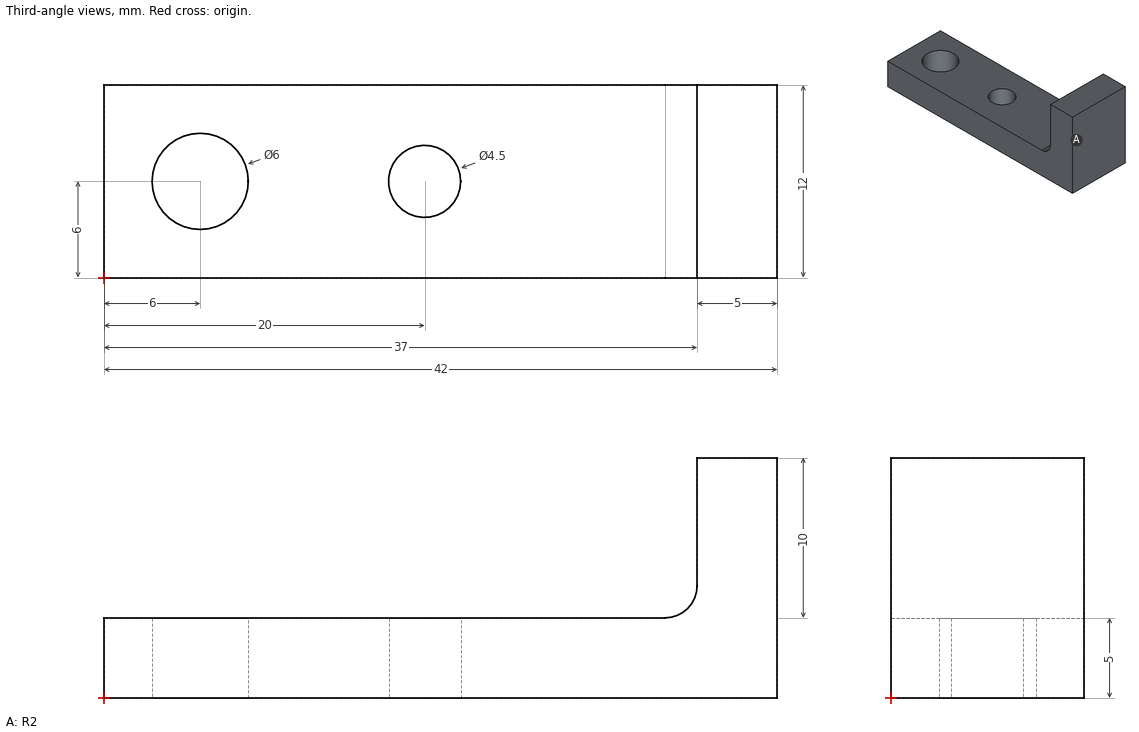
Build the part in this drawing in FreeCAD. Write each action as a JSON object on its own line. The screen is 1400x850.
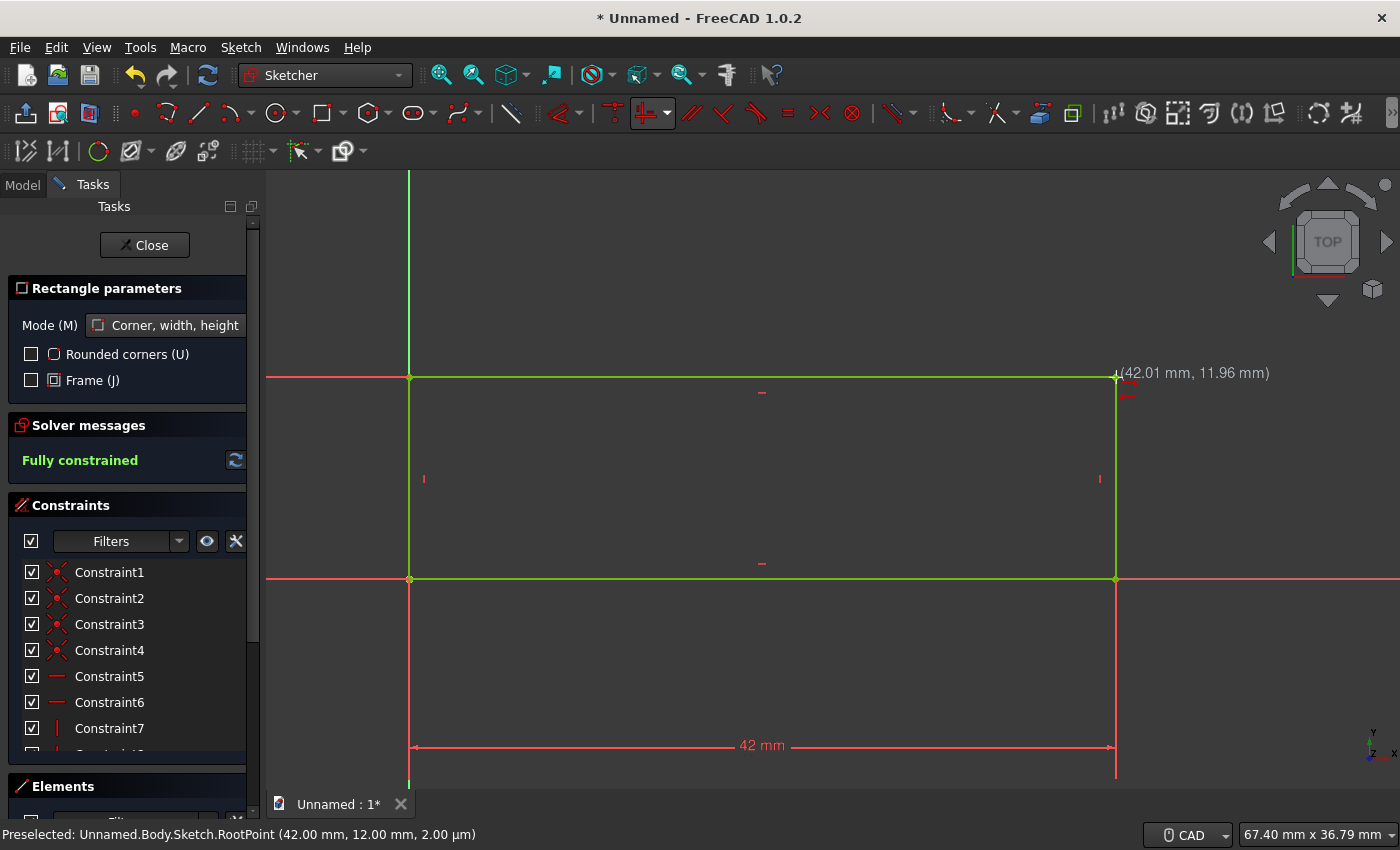
{"action": "left_click", "coordinate": [276, 114]}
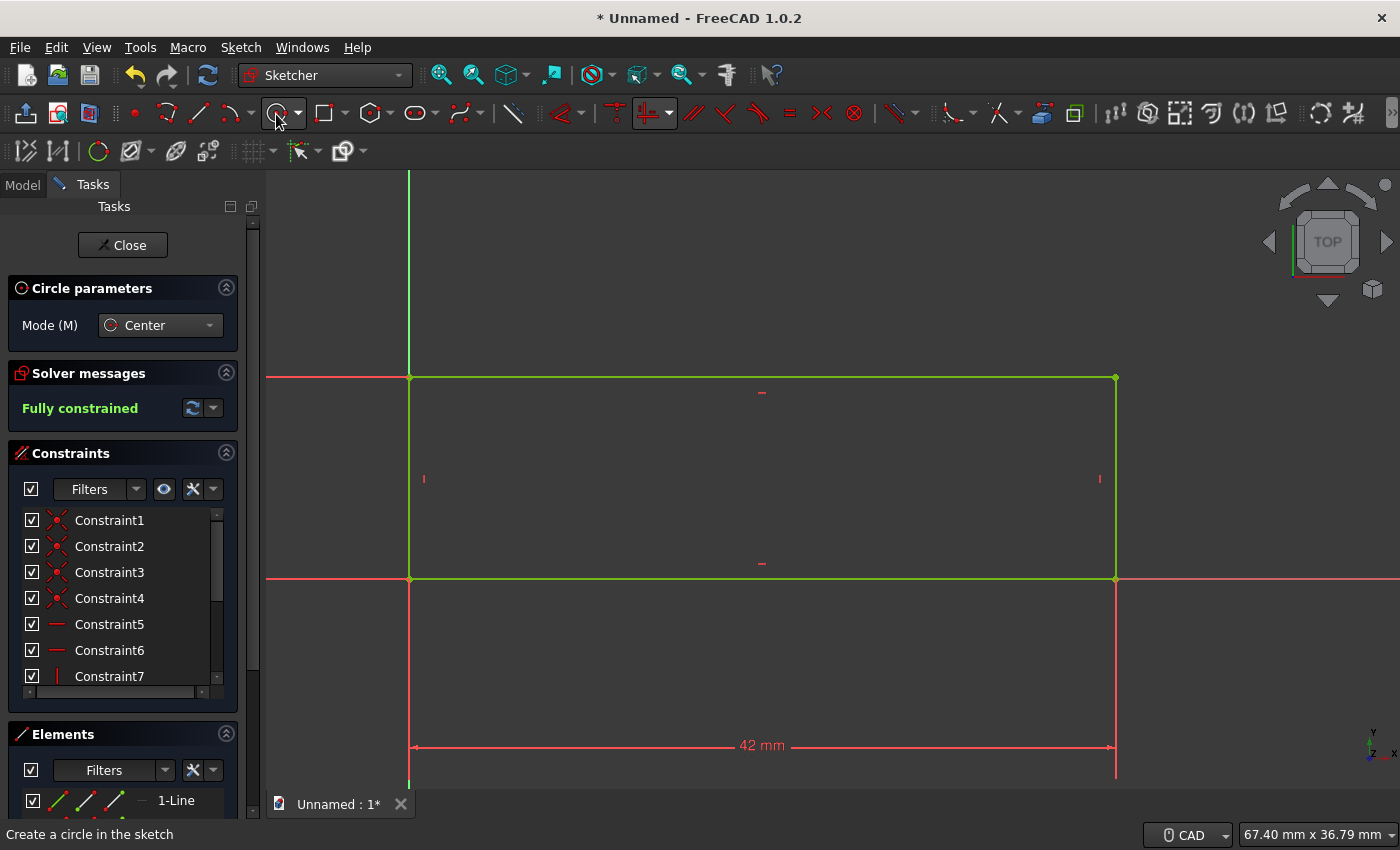
{"action": "left_click", "coordinate": [510, 478]}
{"action": "mouse_move", "coordinate": [546, 443]}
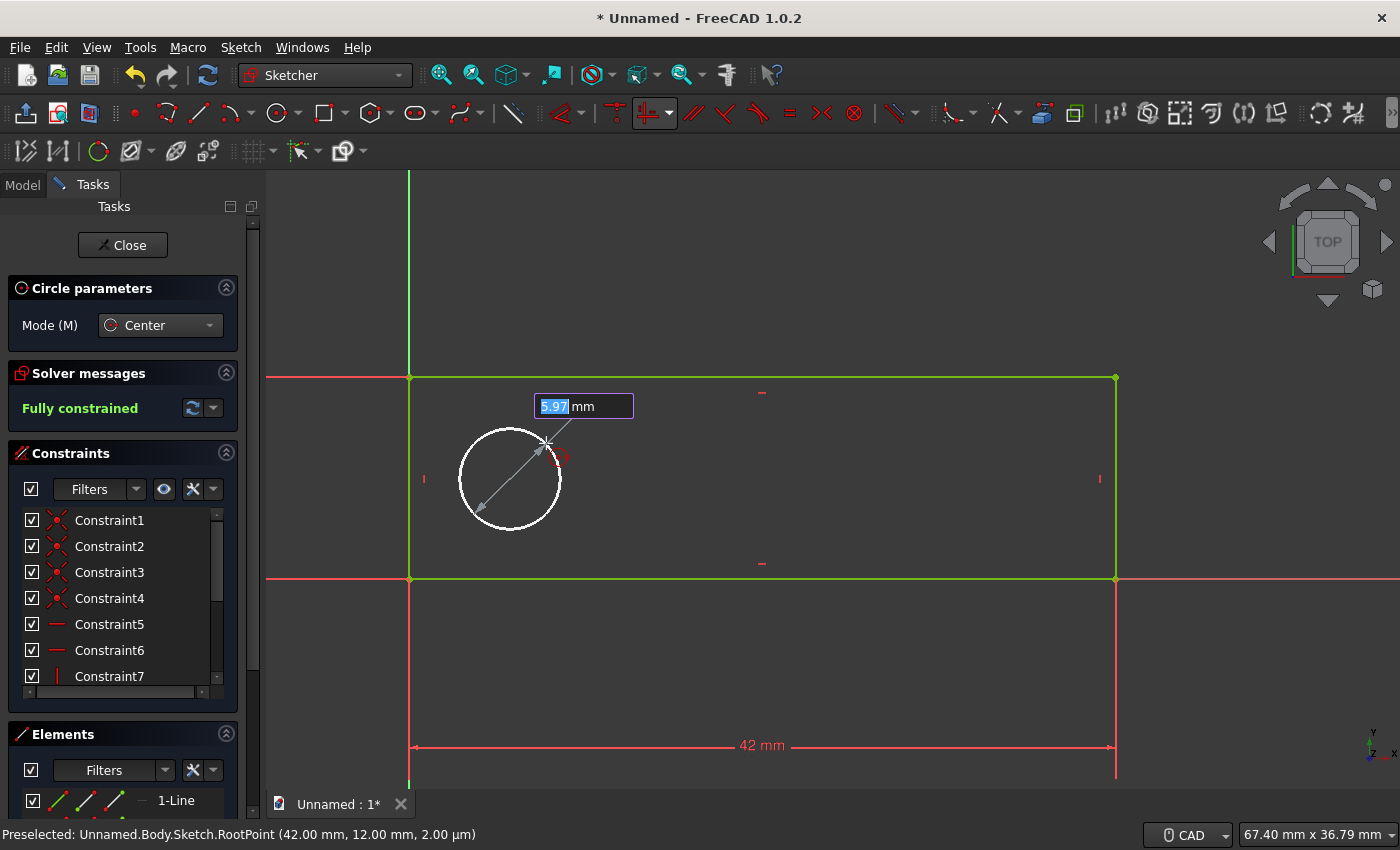
{"action": "type", "text": "6"}
{"action": "key", "text": "Return"}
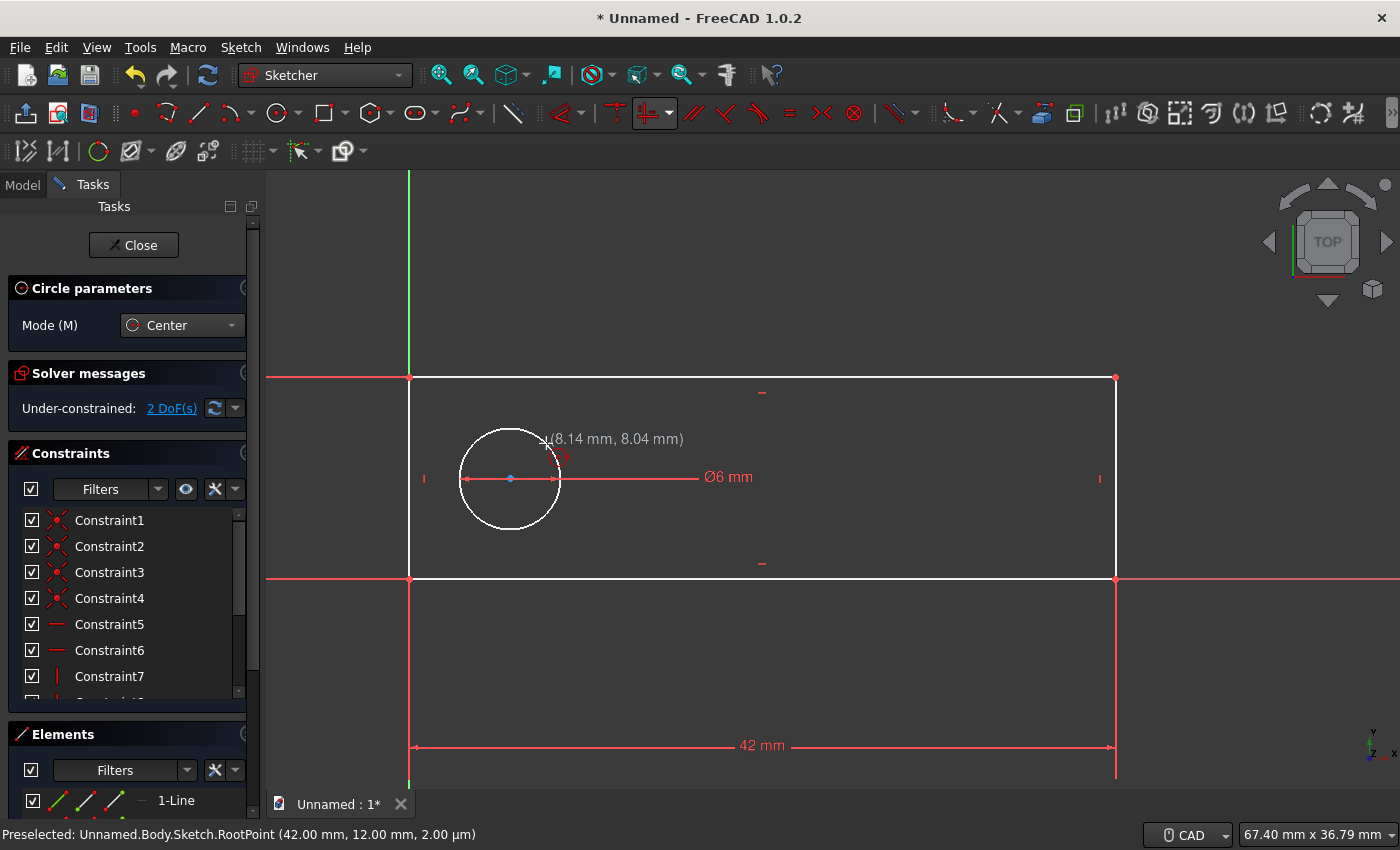
{"action": "left_click", "coordinate": [746, 478]}
{"action": "mouse_move", "coordinate": [772, 452]}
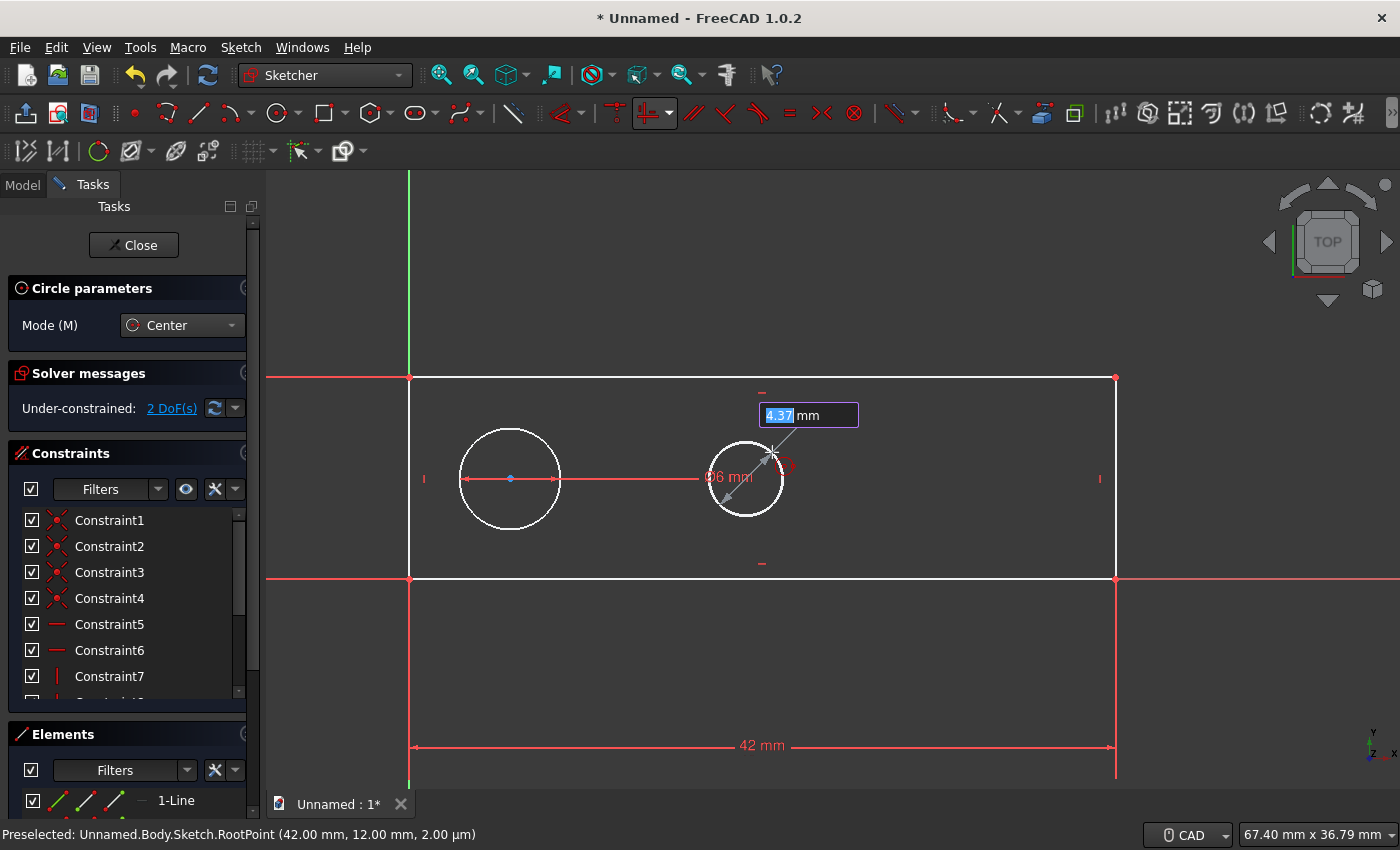
{"action": "type", "text": "4.5"}
{"action": "key", "text": "Return"}
{"action": "key", "text": "Escape"}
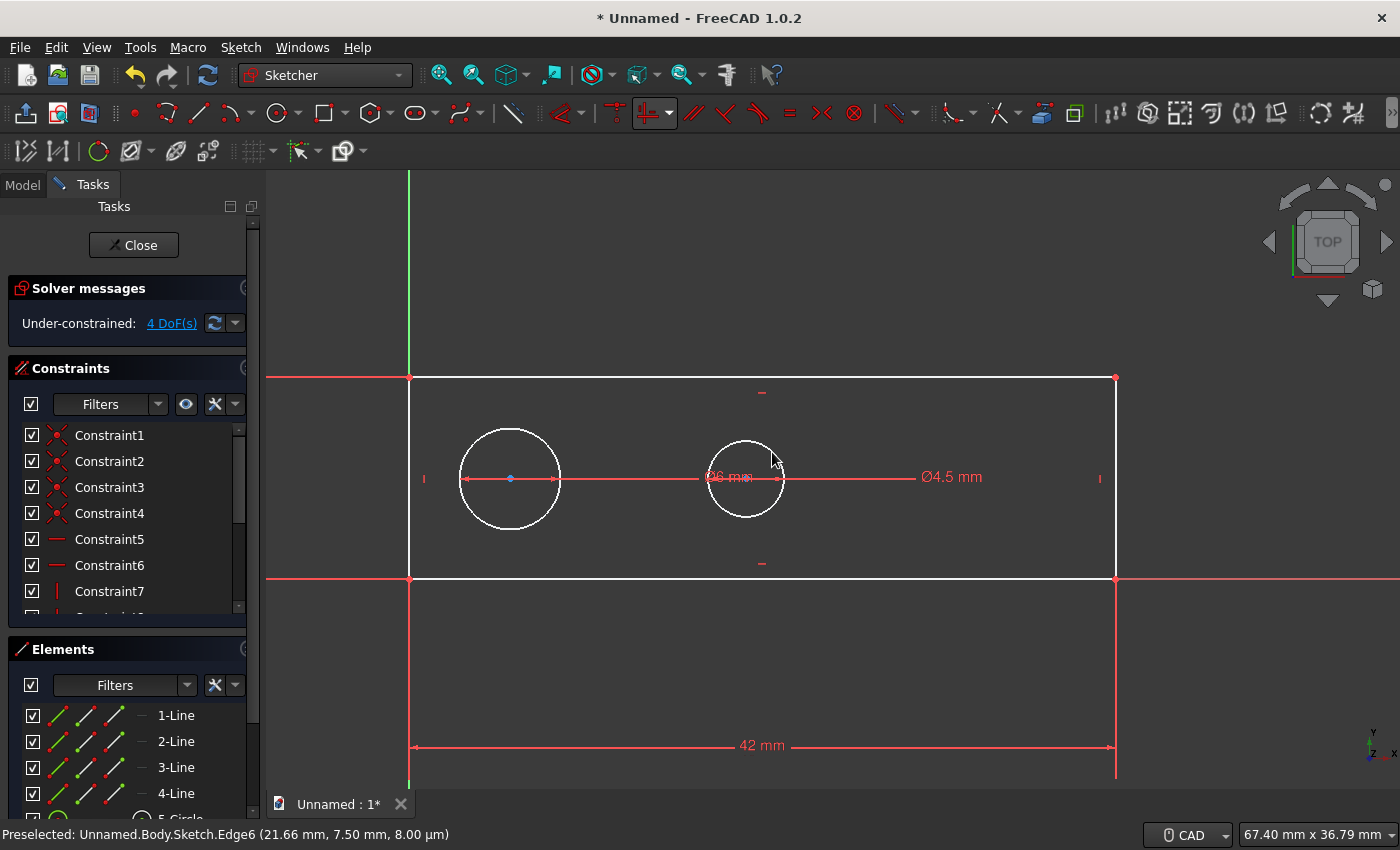
{"action": "left_click", "coordinate": [510, 479]}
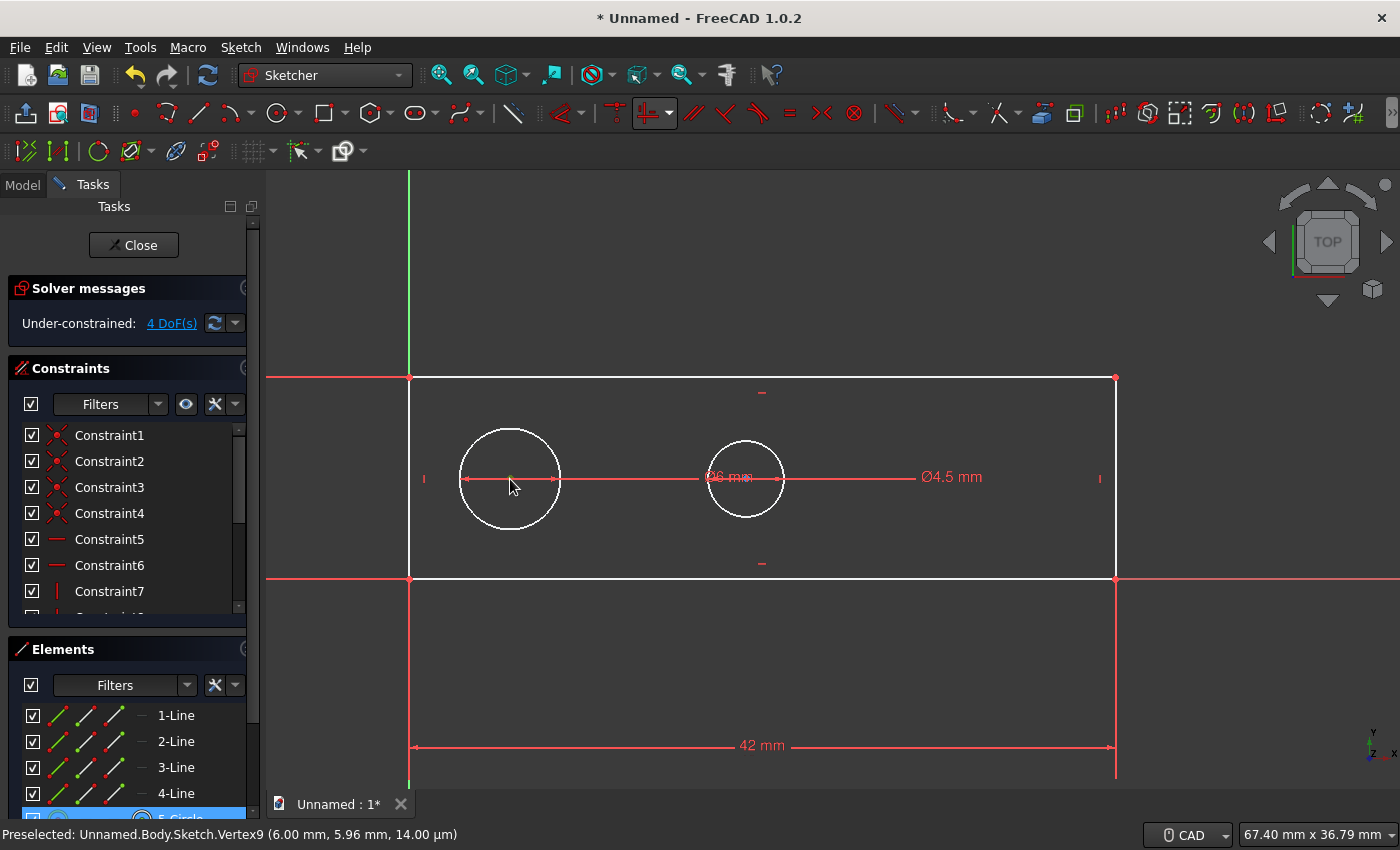
{"action": "left_click", "coordinate": [746, 479]}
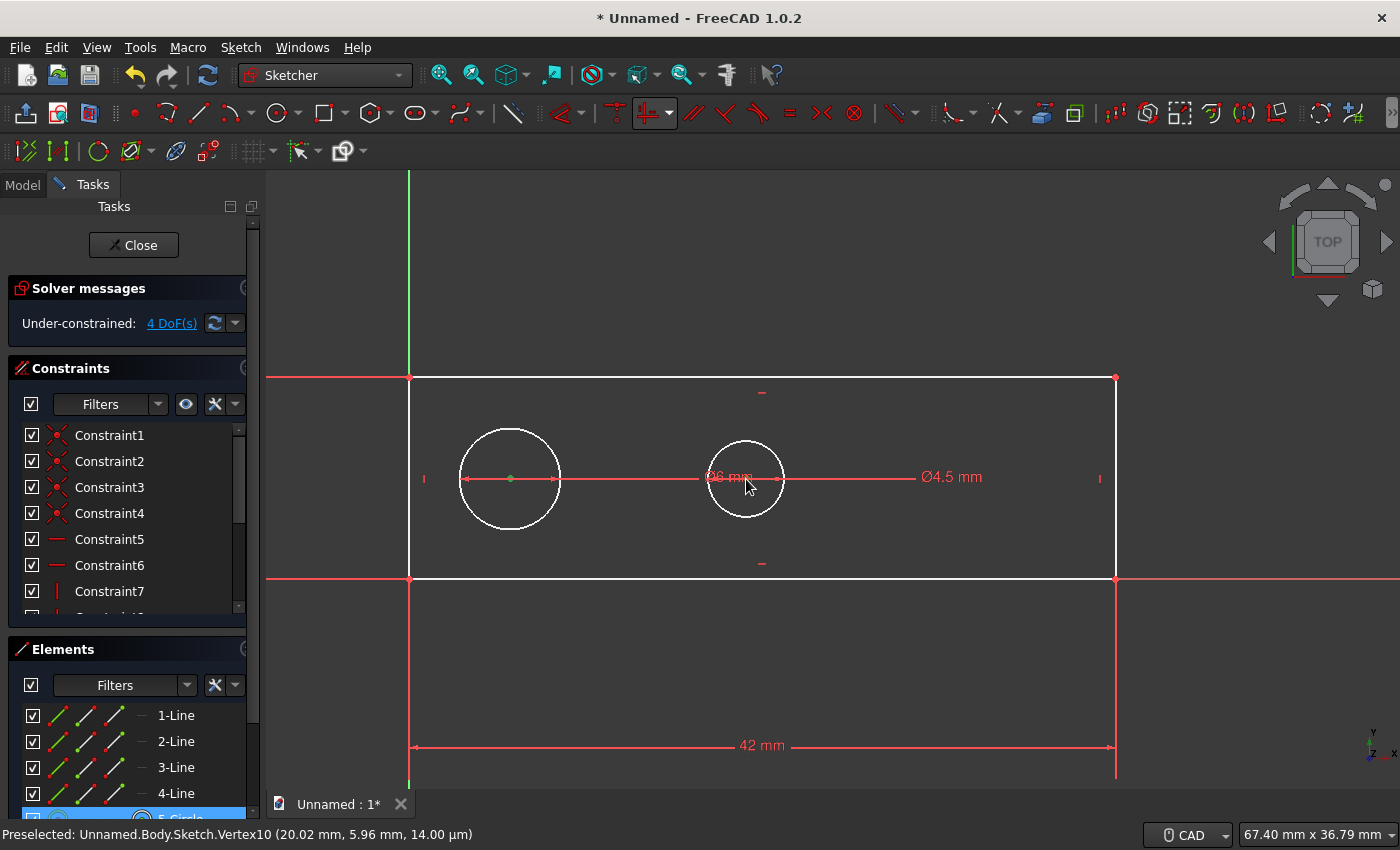
{"action": "left_click", "coordinate": [672, 114]}